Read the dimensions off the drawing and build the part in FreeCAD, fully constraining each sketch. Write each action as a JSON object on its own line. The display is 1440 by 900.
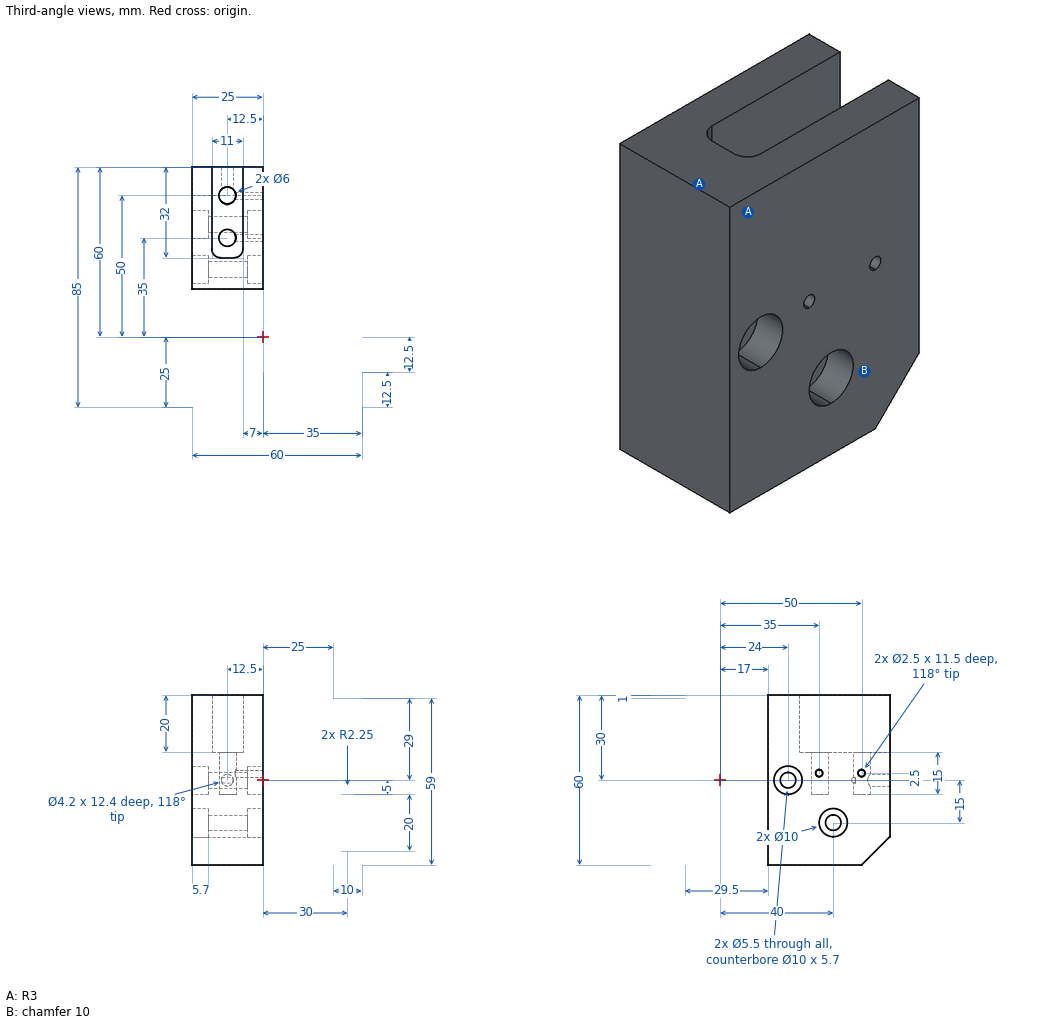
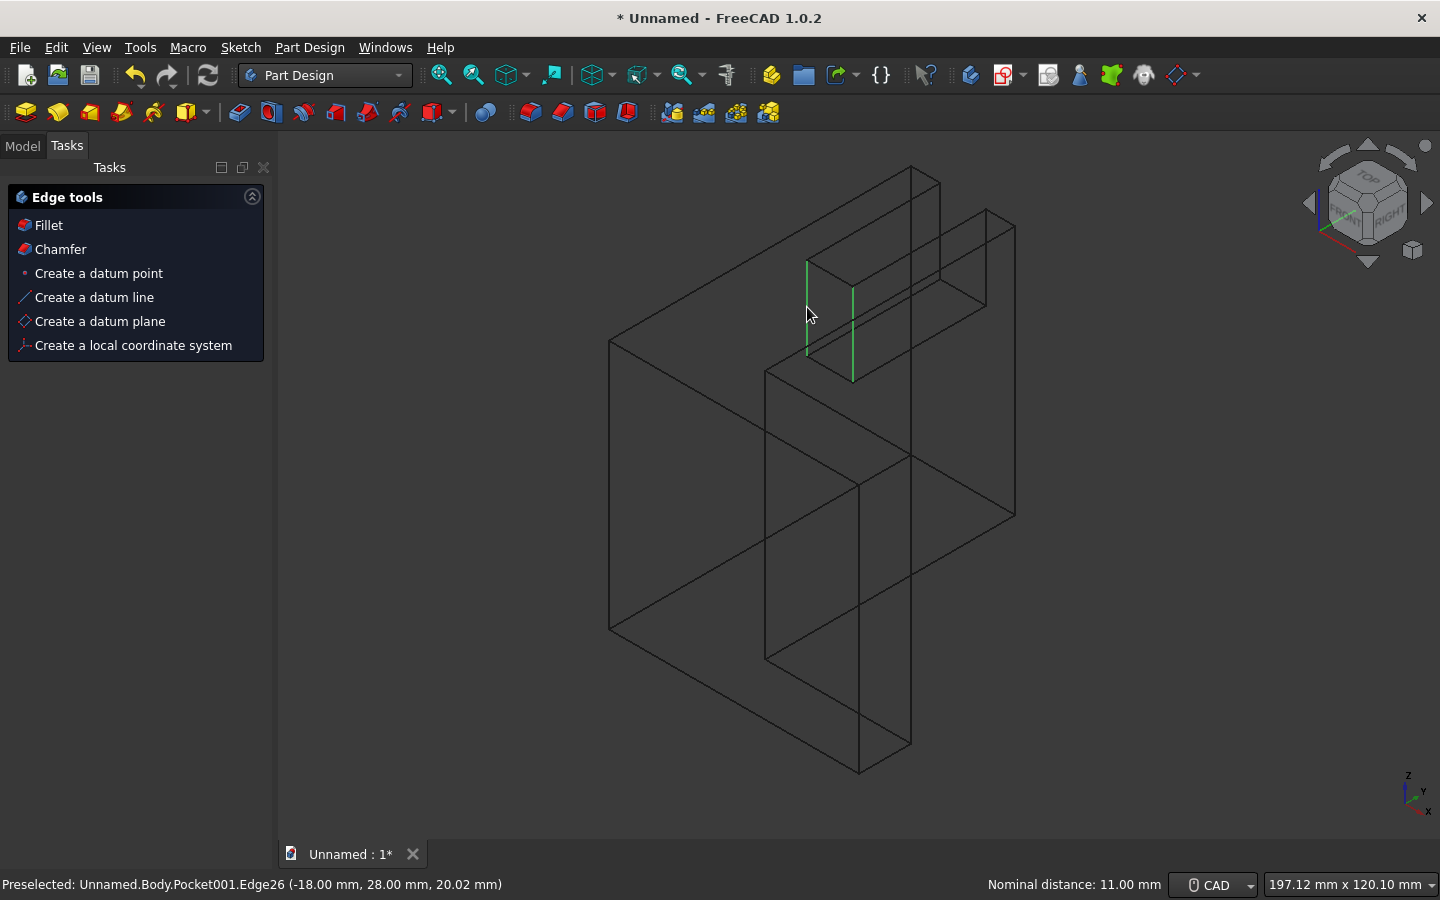
{"action": "key", "text": "v 1"}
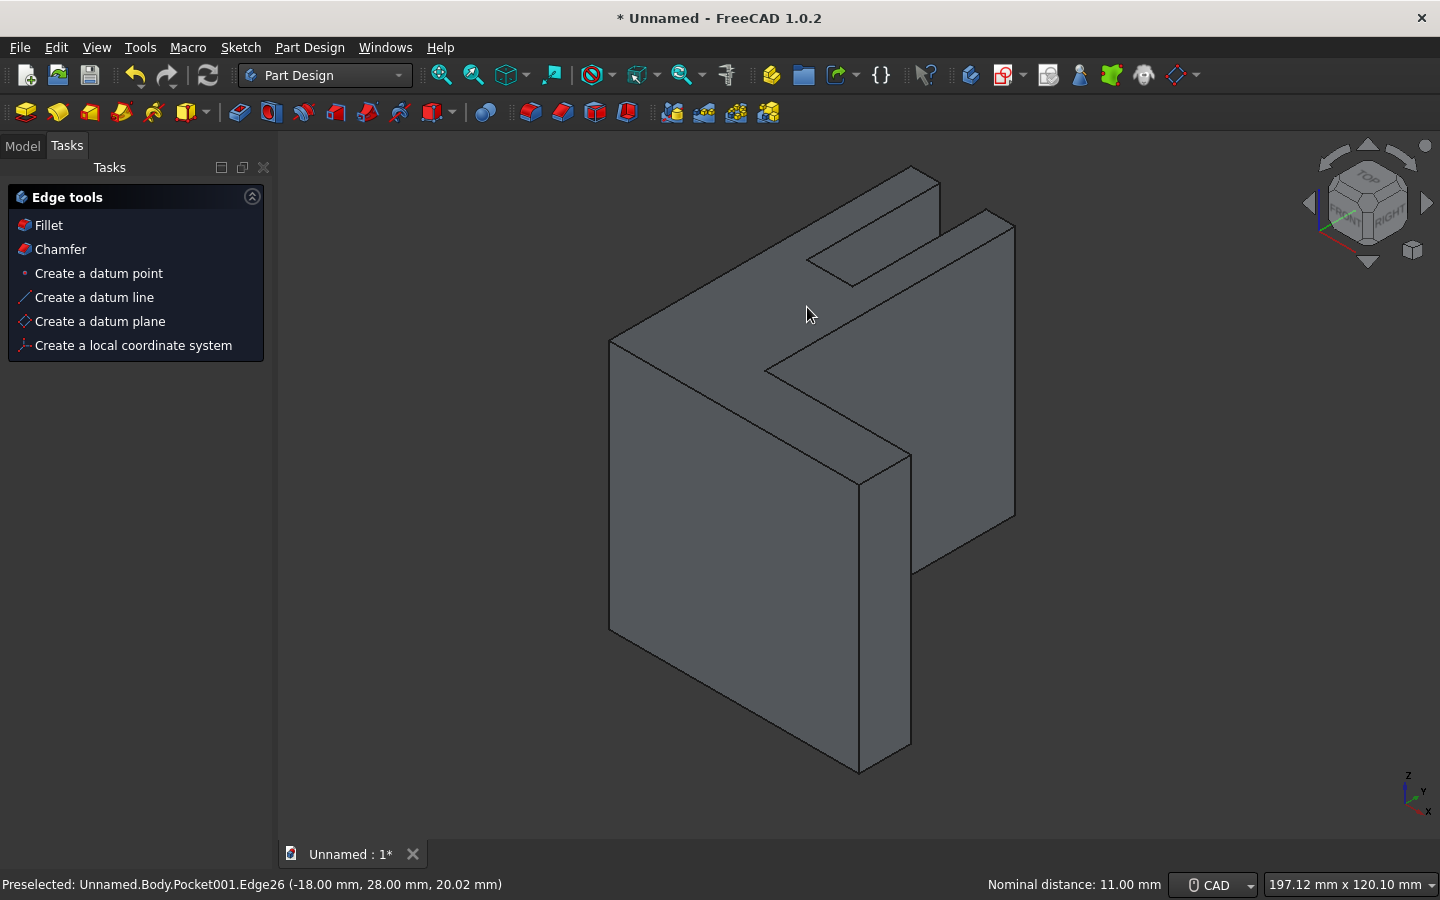
{"action": "left_click", "coordinate": [532, 112]}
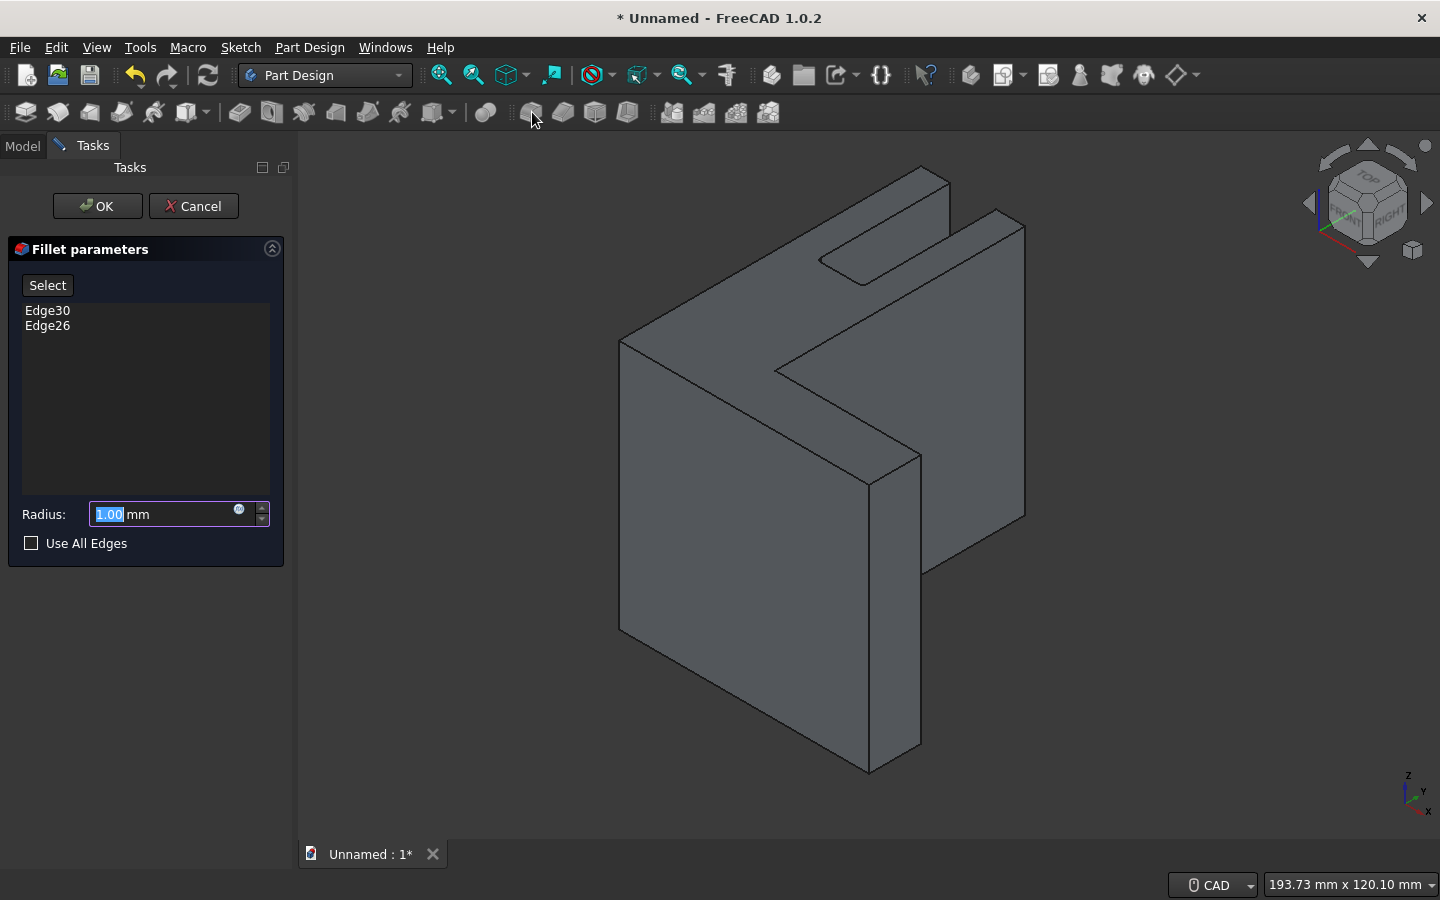
{"action": "type", "text": "3"}
{"action": "key", "text": "Tab"}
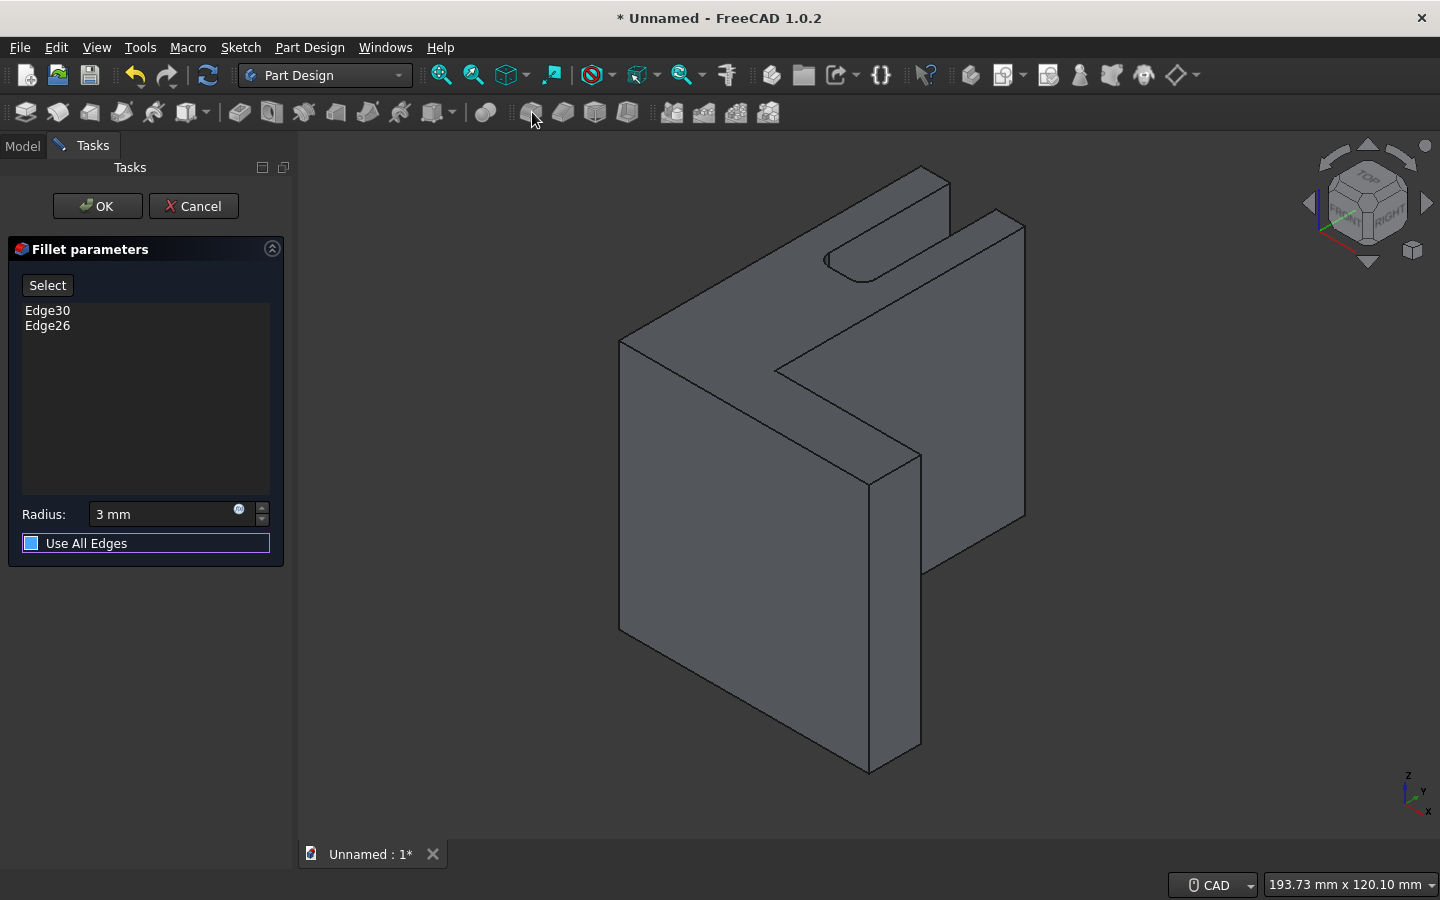
{"action": "left_click", "coordinate": [98, 206]}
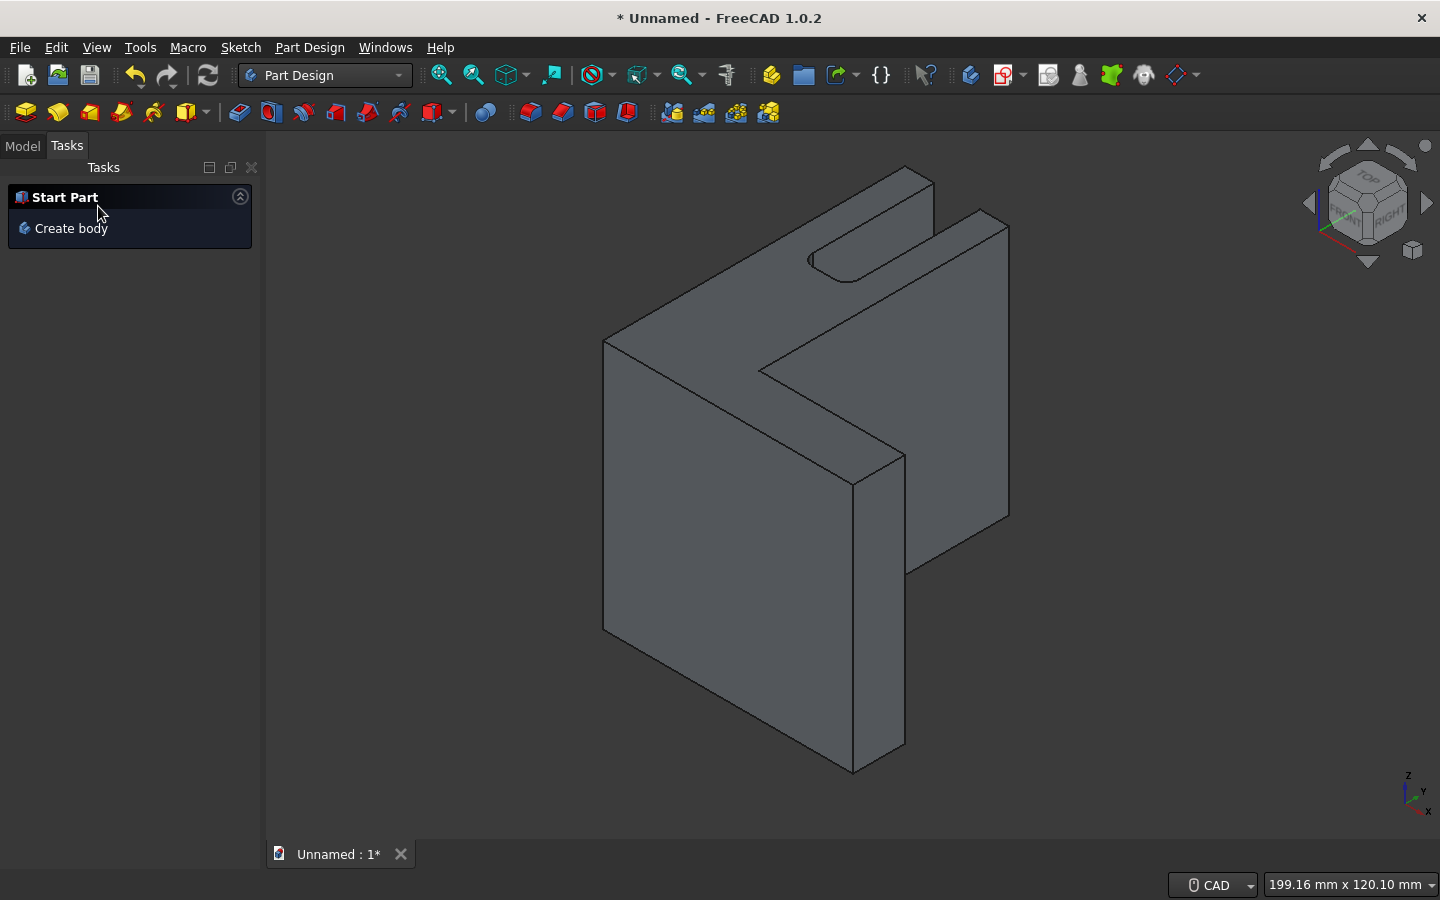
{"action": "key", "text": "2"}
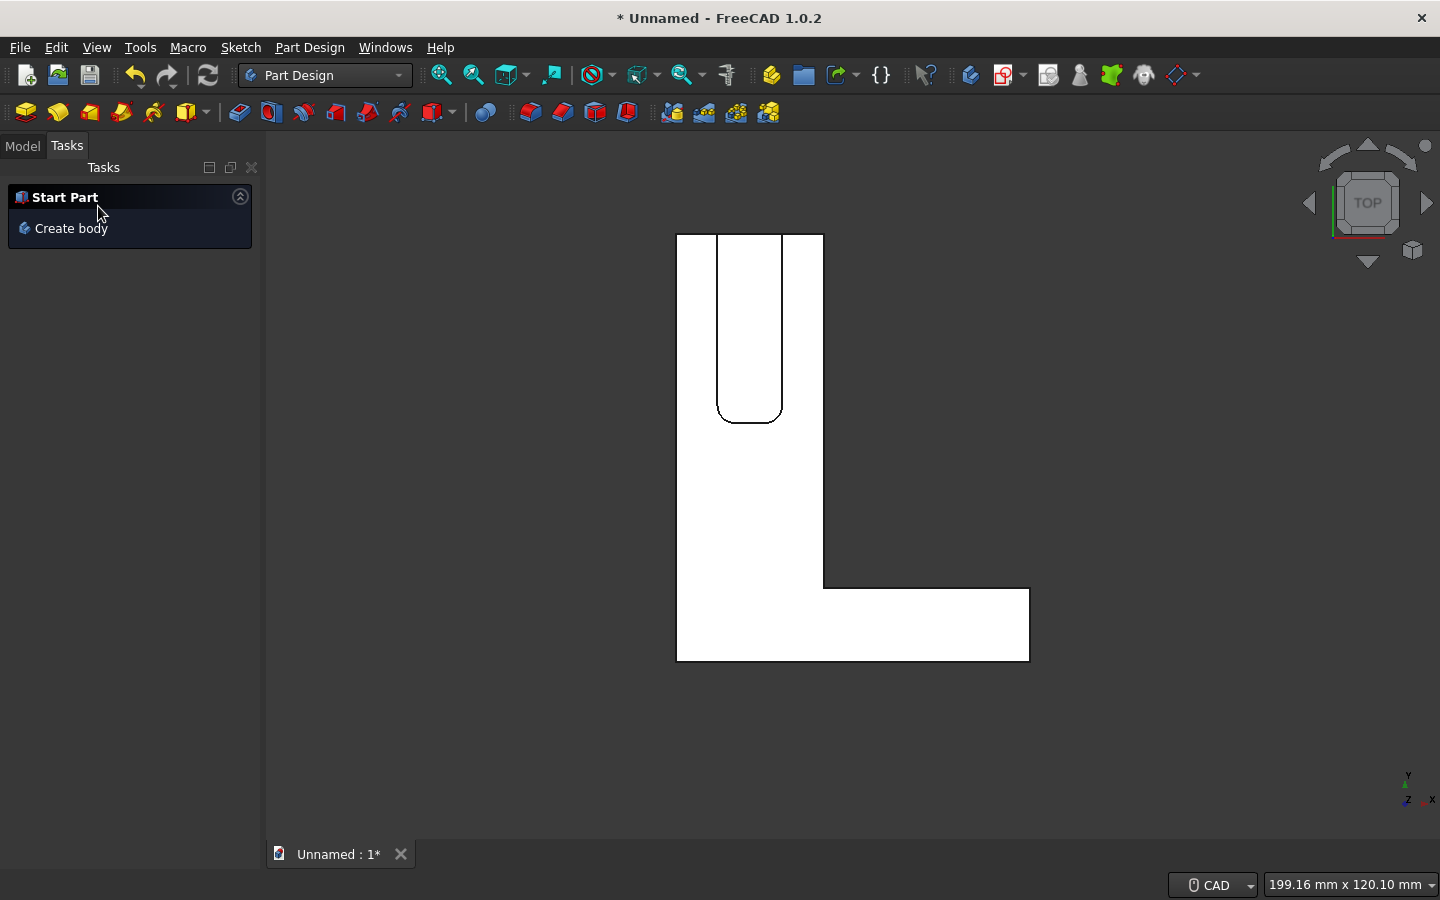
{"action": "left_click", "coordinate": [750, 274]}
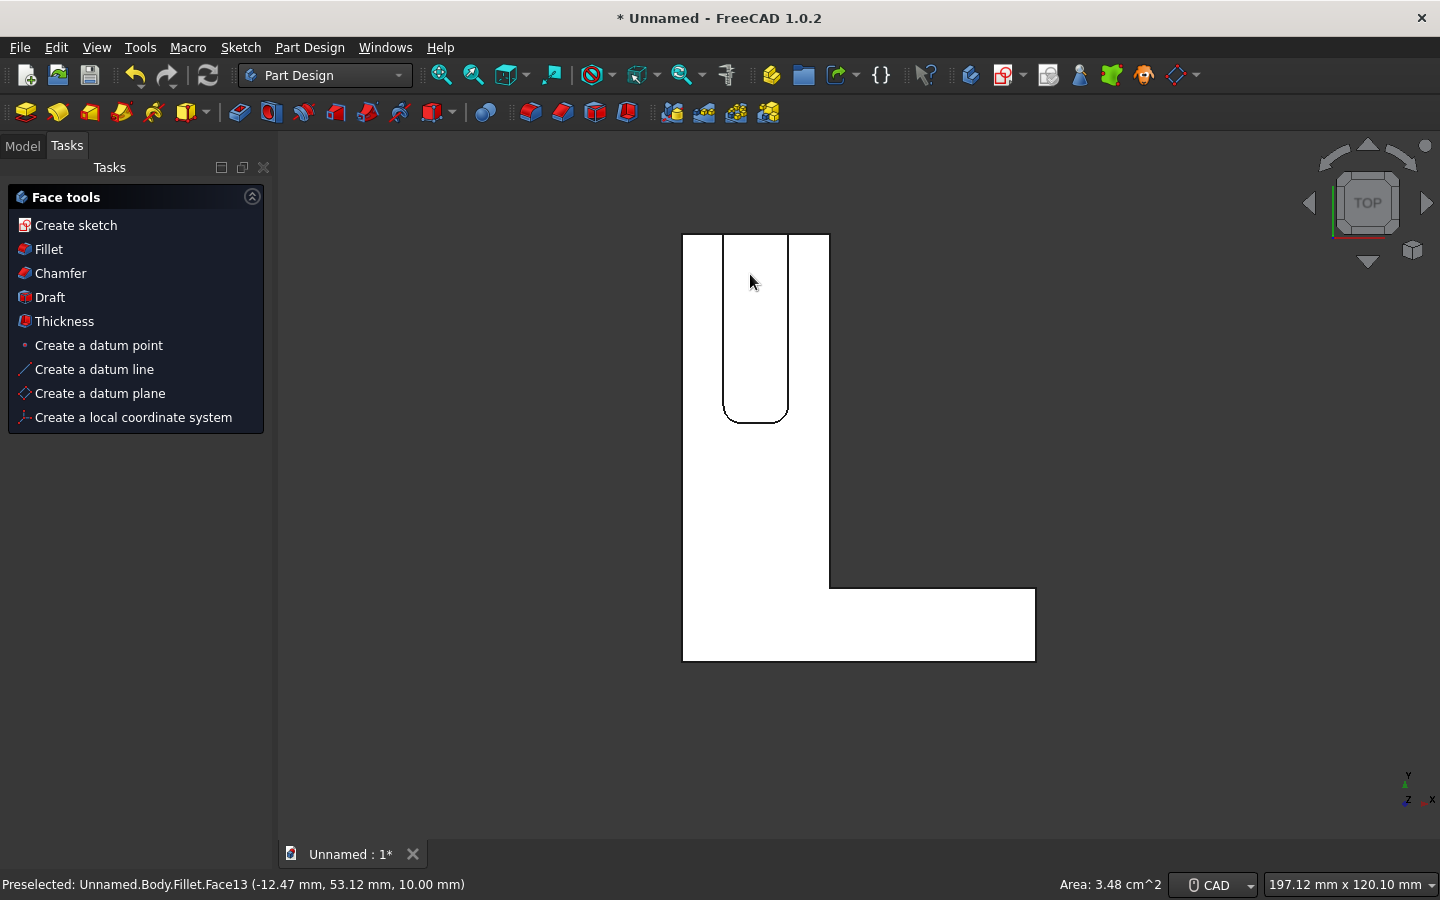
{"action": "left_click", "coordinate": [1004, 76]}